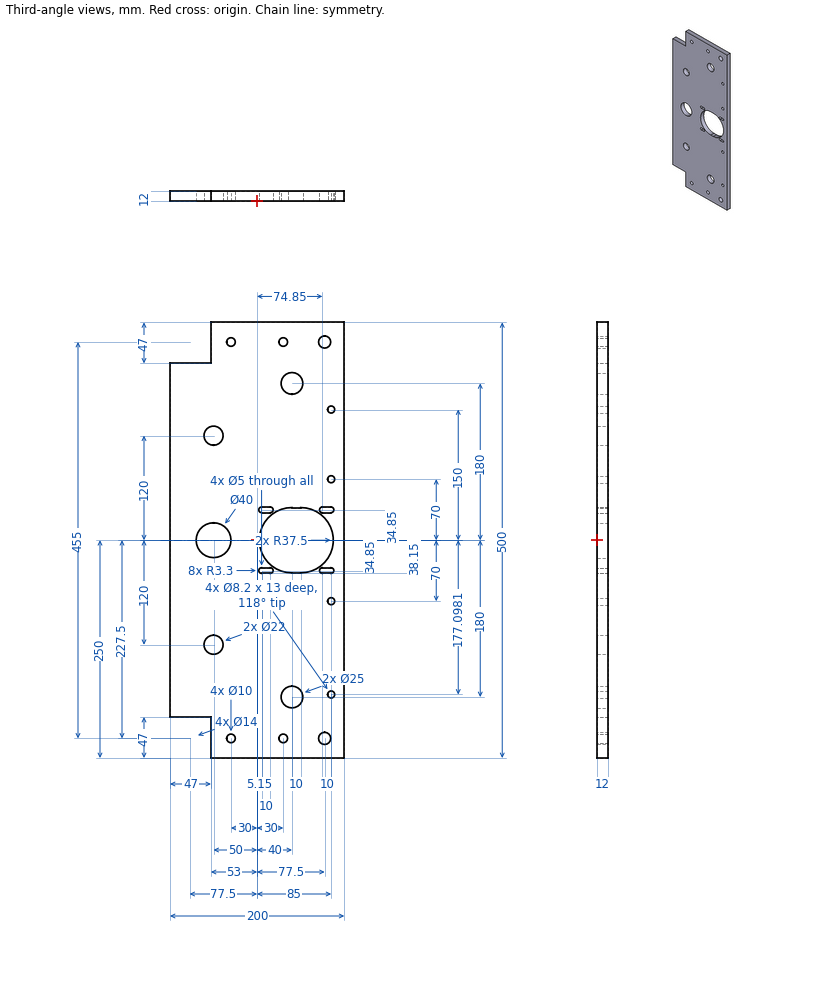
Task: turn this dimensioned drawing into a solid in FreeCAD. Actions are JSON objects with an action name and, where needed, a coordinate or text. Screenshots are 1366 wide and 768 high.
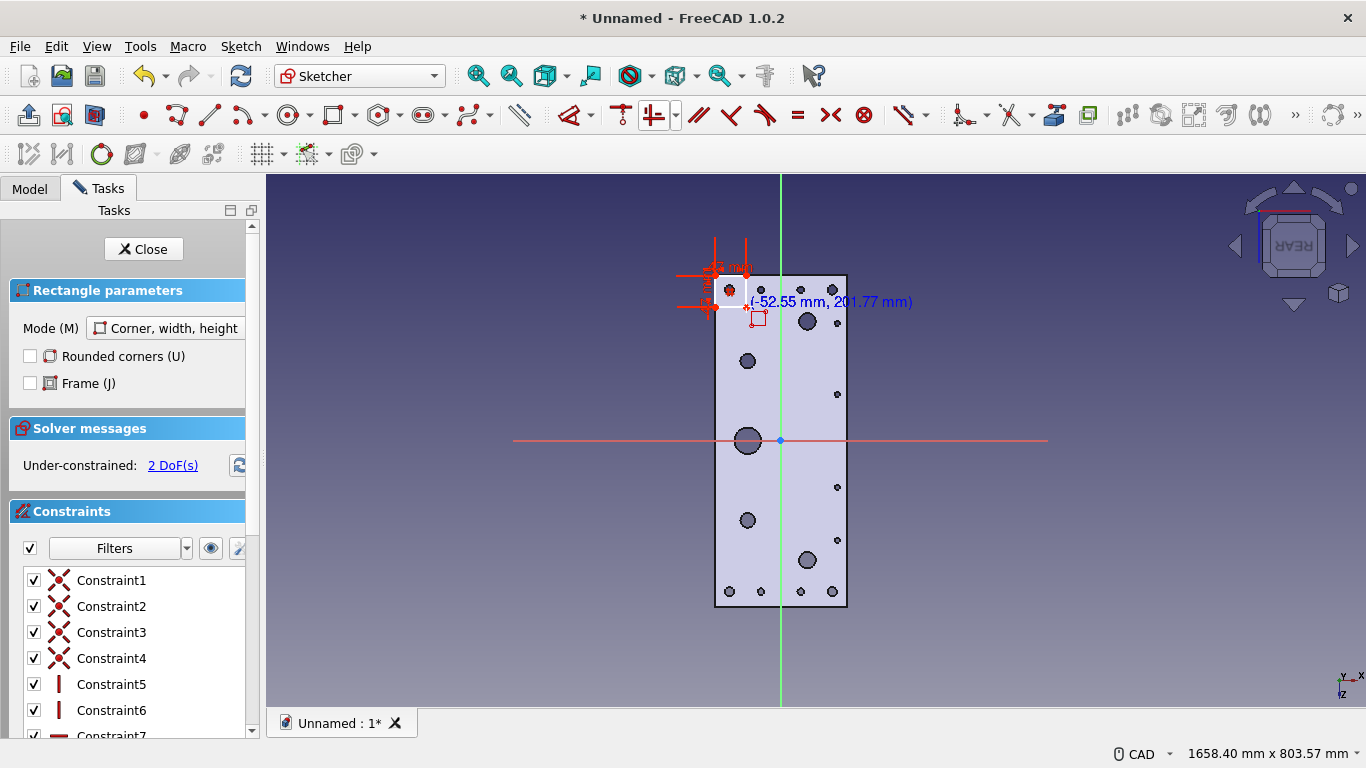
{"action": "left_click", "coordinate": [715, 575]}
{"action": "mouse_move", "coordinate": [746, 607]}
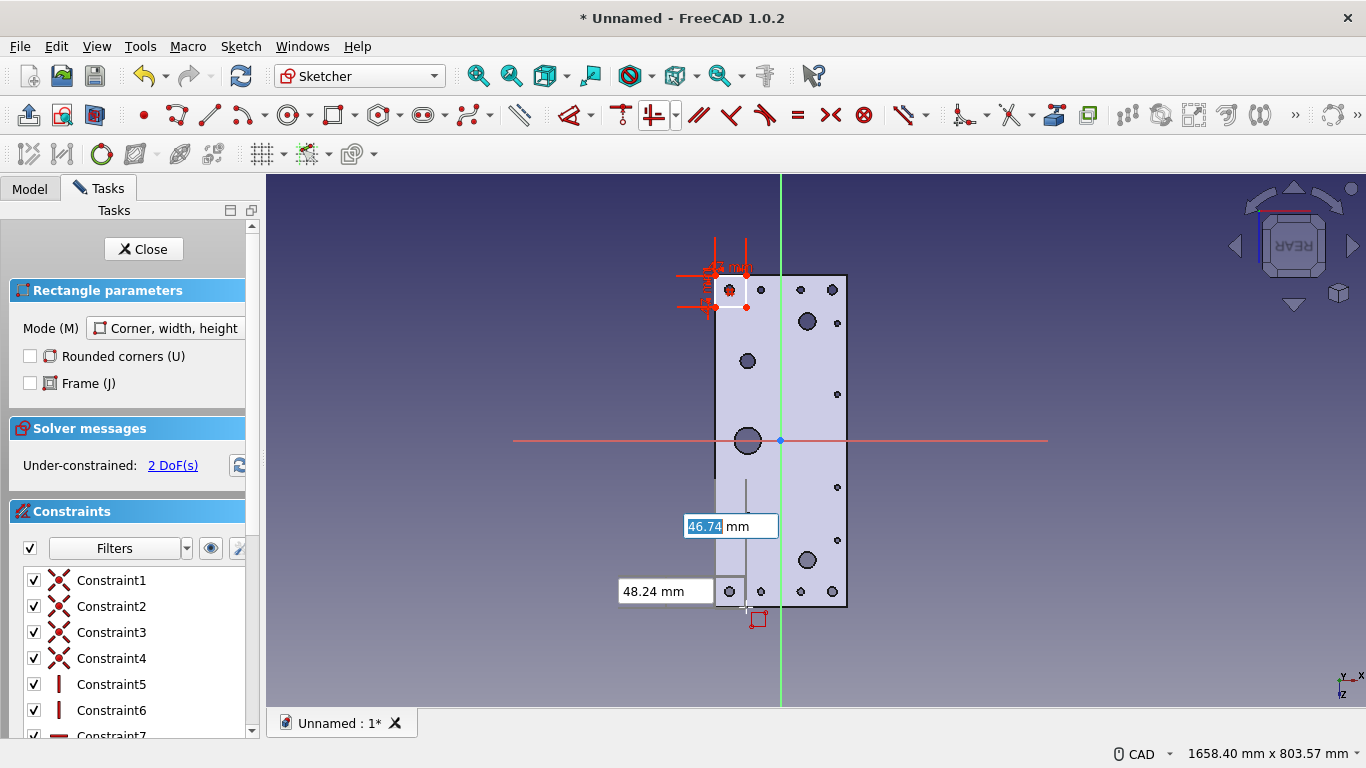
{"action": "type", "text": "47"}
{"action": "key", "text": "Tab"}
{"action": "type", "text": "47"}
{"action": "key", "text": "Return"}
{"action": "key", "text": "Escape"}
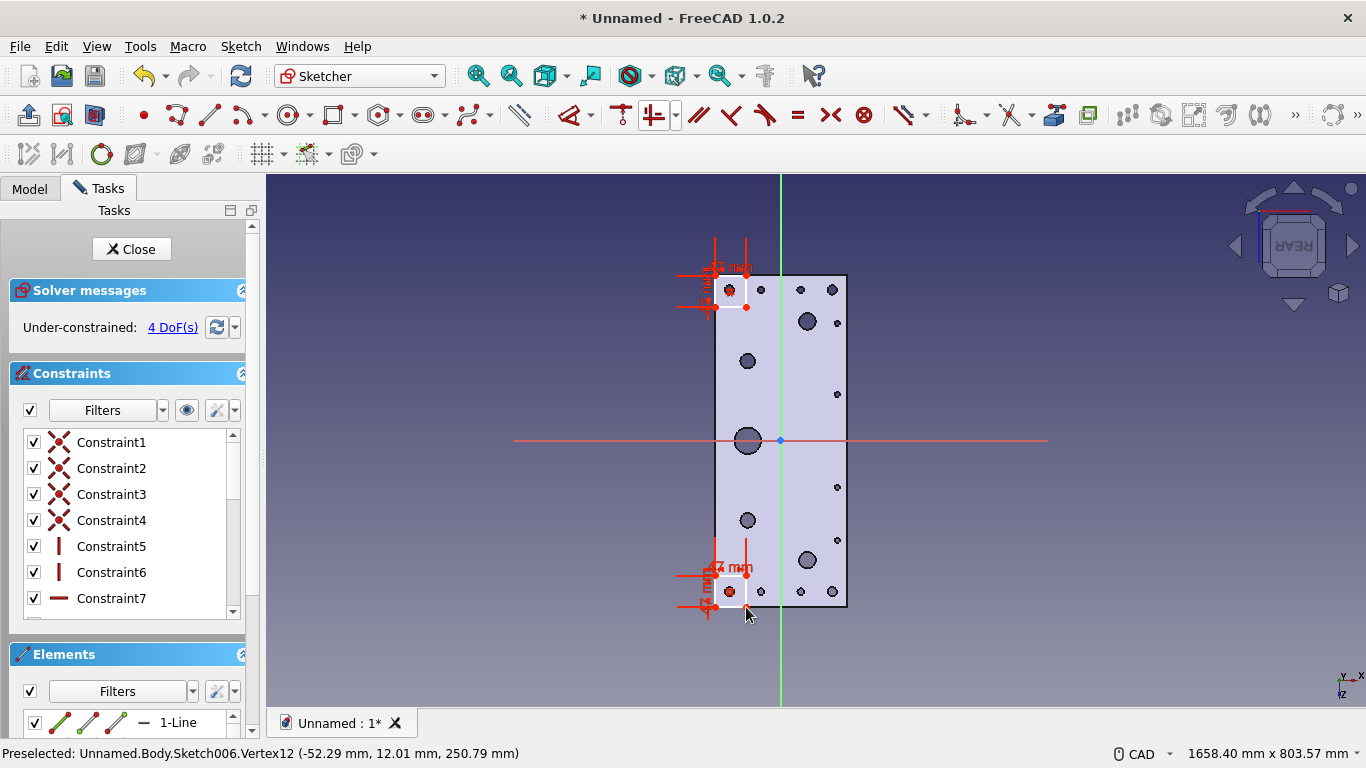
{"action": "left_click", "coordinate": [715, 307]}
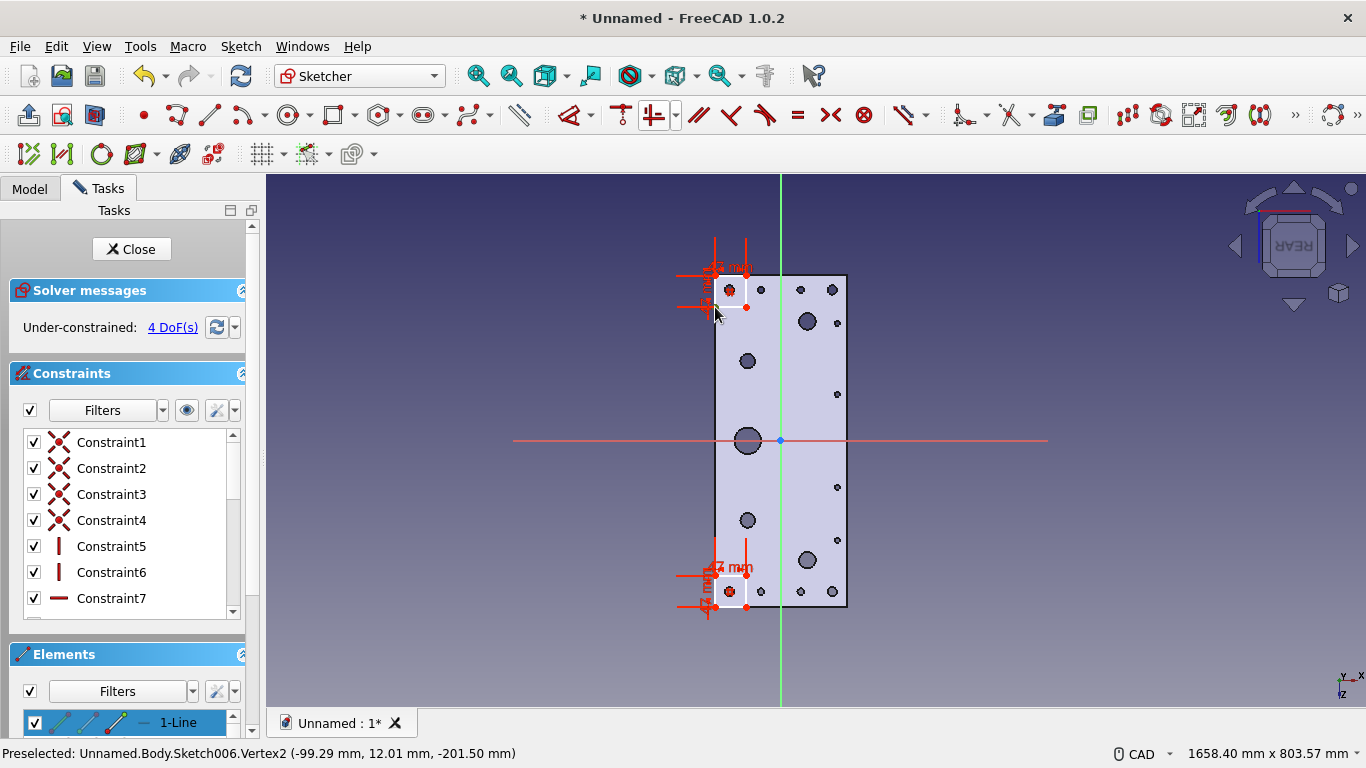
{"action": "left_click", "coordinate": [715, 576]}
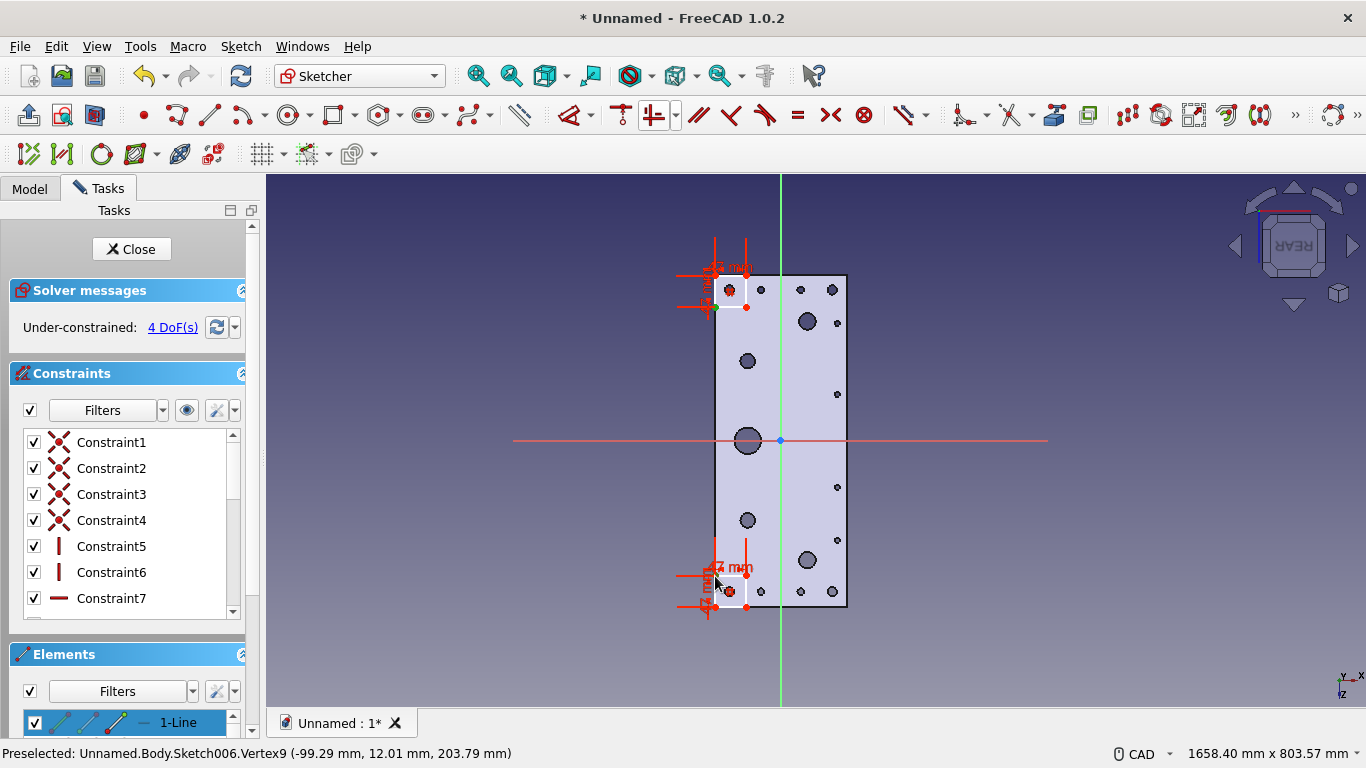
{"action": "left_click", "coordinate": [553, 441]}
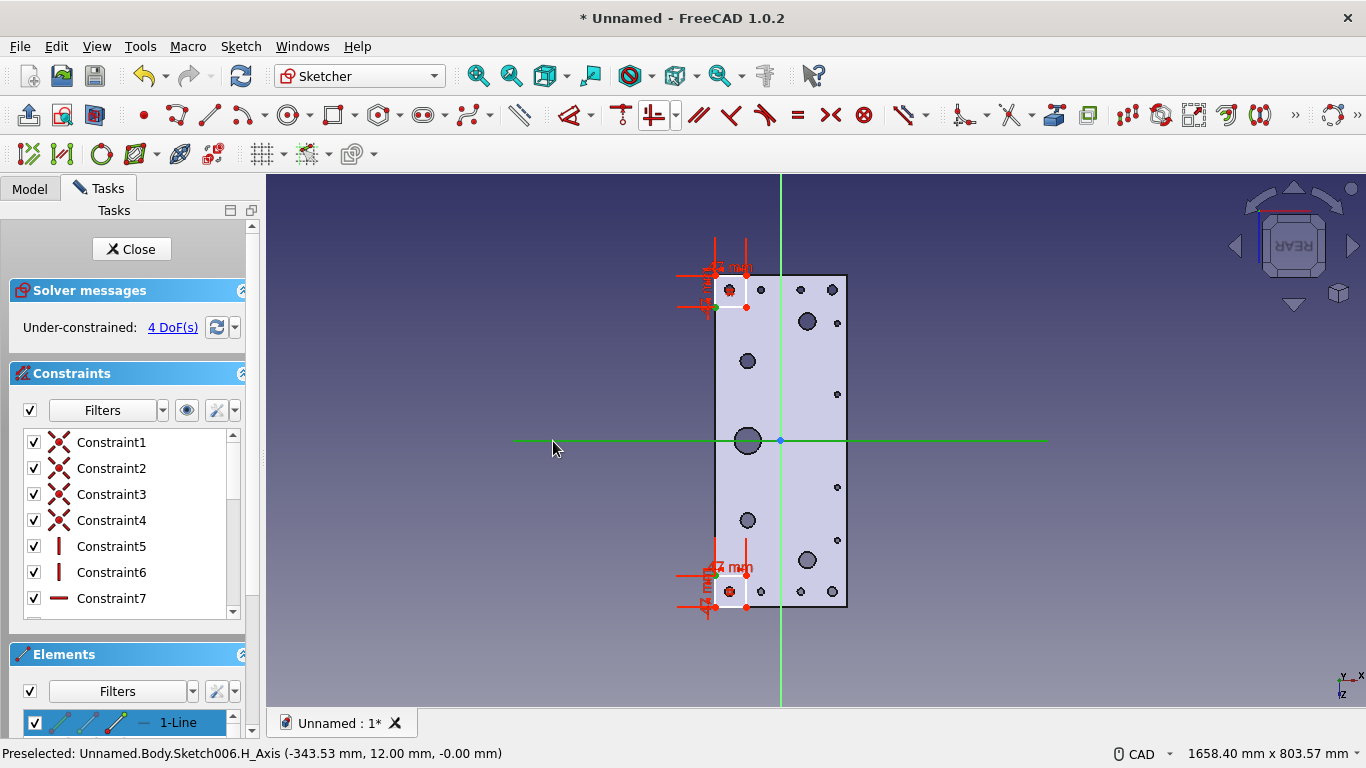
{"action": "key", "text": "s"}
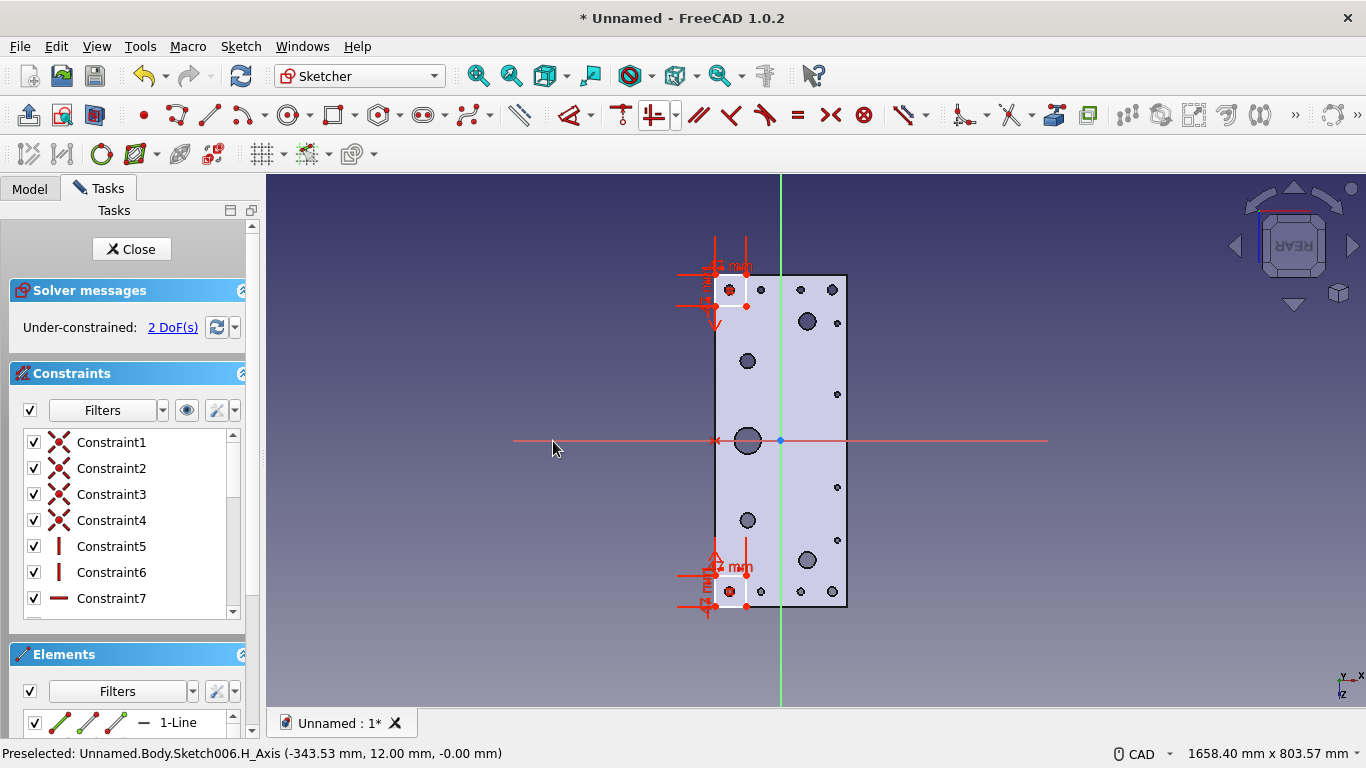
{"action": "key", "text": "d"}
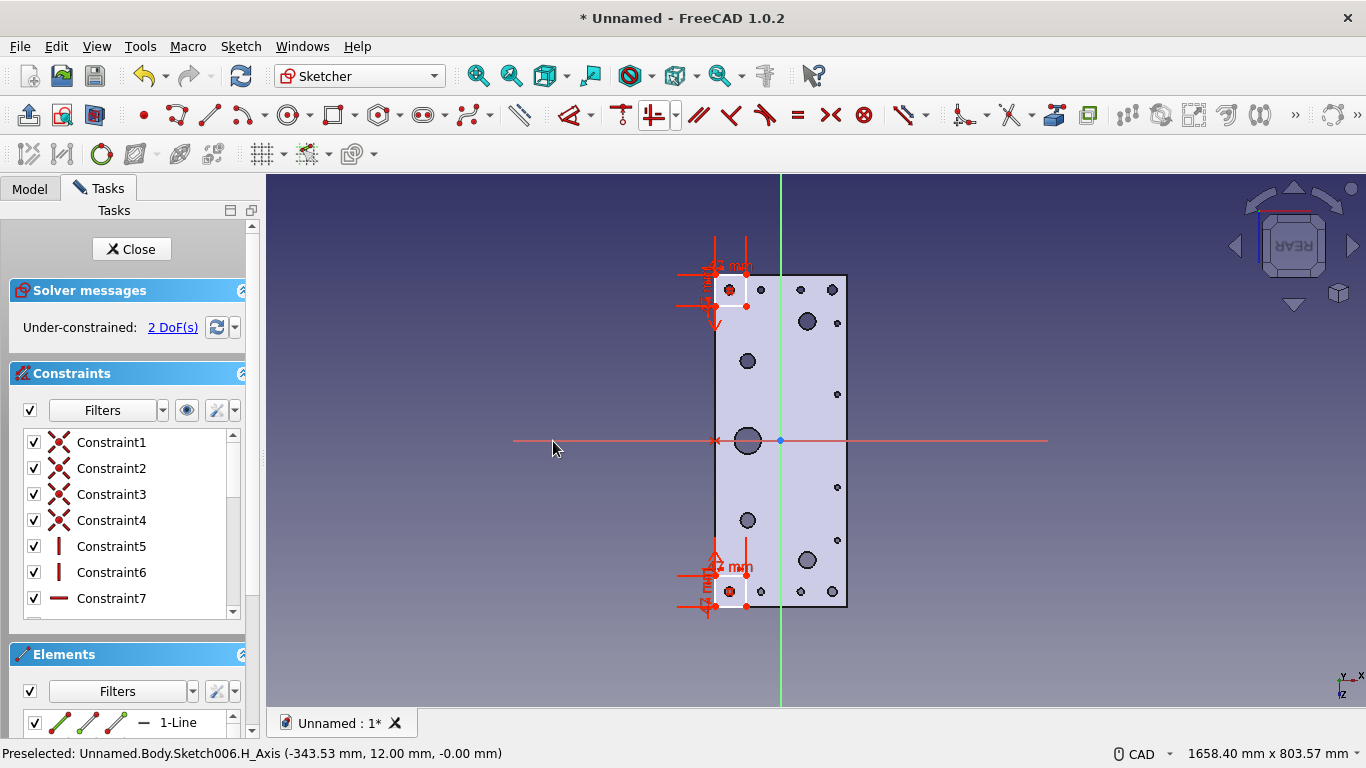
{"action": "left_click", "coordinate": [746, 306]}
{"action": "left_click", "coordinate": [764, 272]}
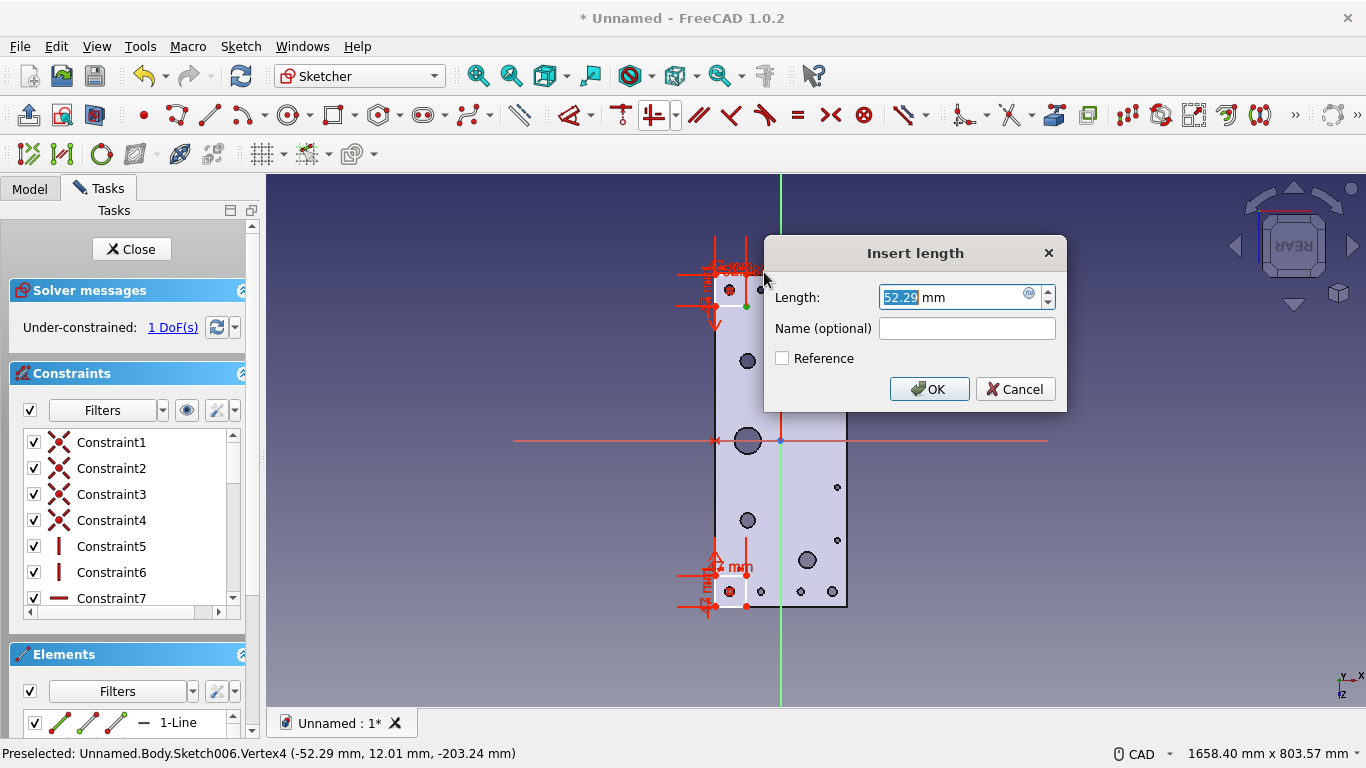
{"action": "type", "text": "53"}
{"action": "key", "text": "Return"}